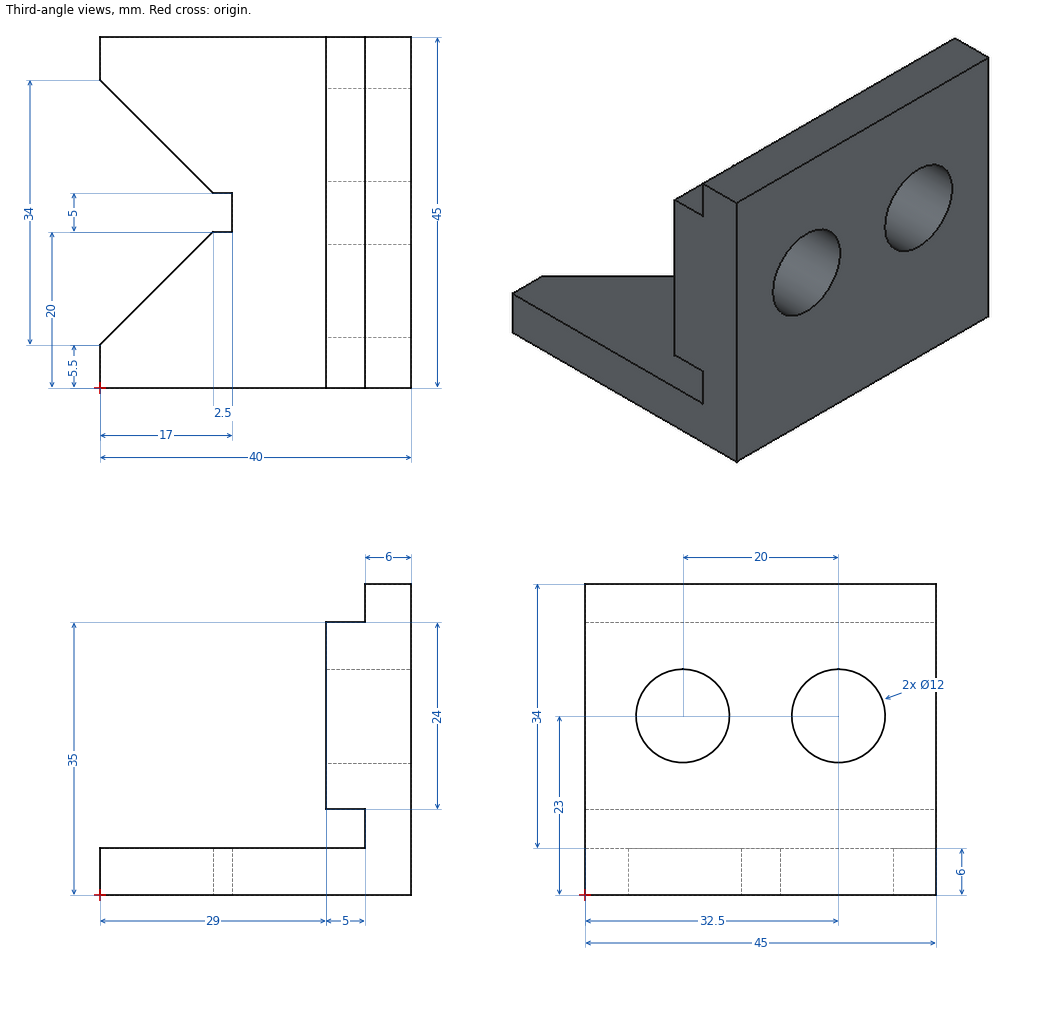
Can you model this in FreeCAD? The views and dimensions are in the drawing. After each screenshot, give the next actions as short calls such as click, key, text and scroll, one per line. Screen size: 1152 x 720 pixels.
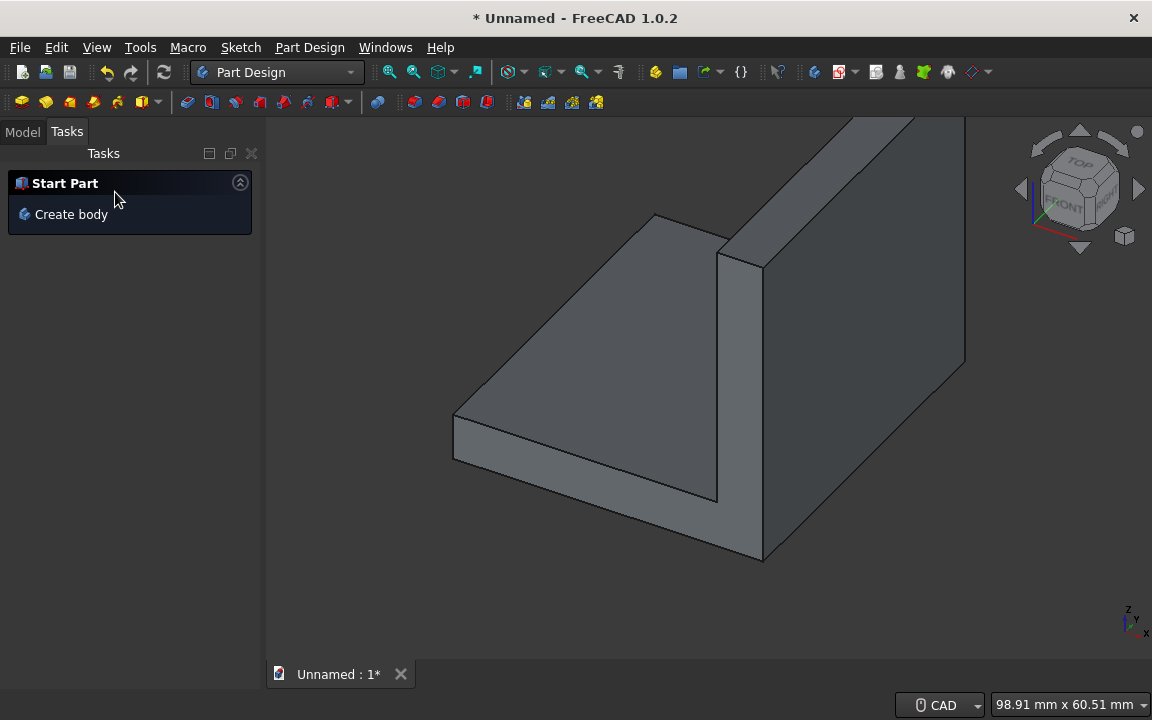
click(390, 72)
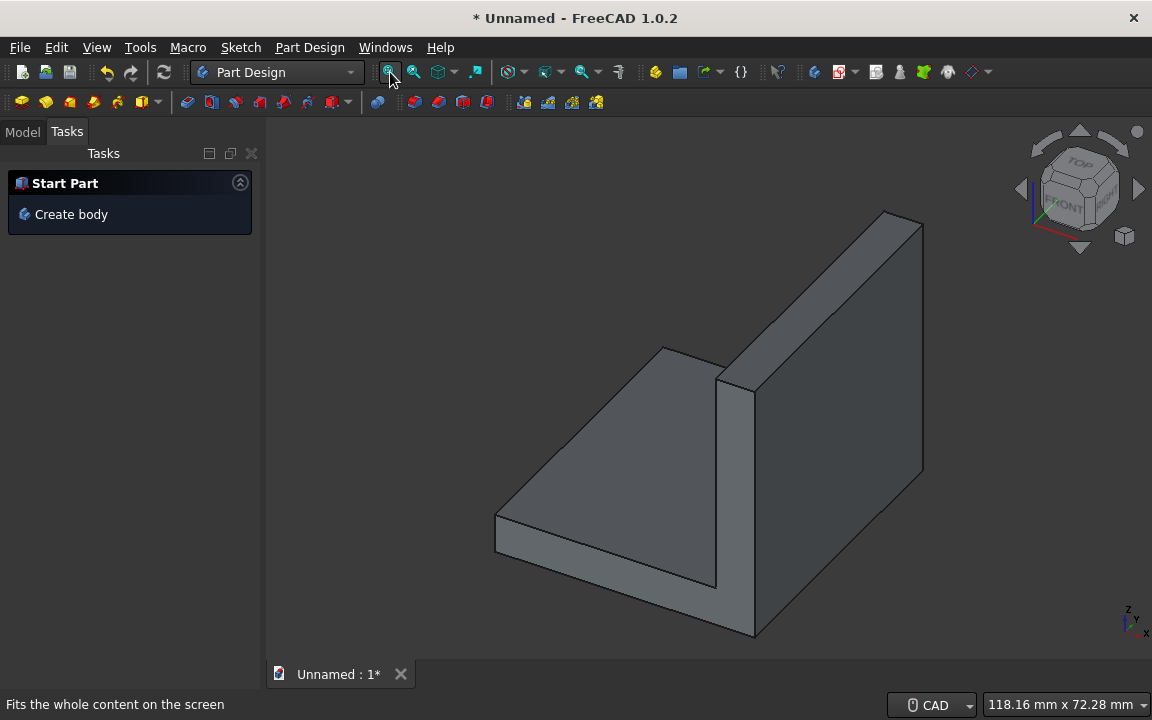
click(840, 72)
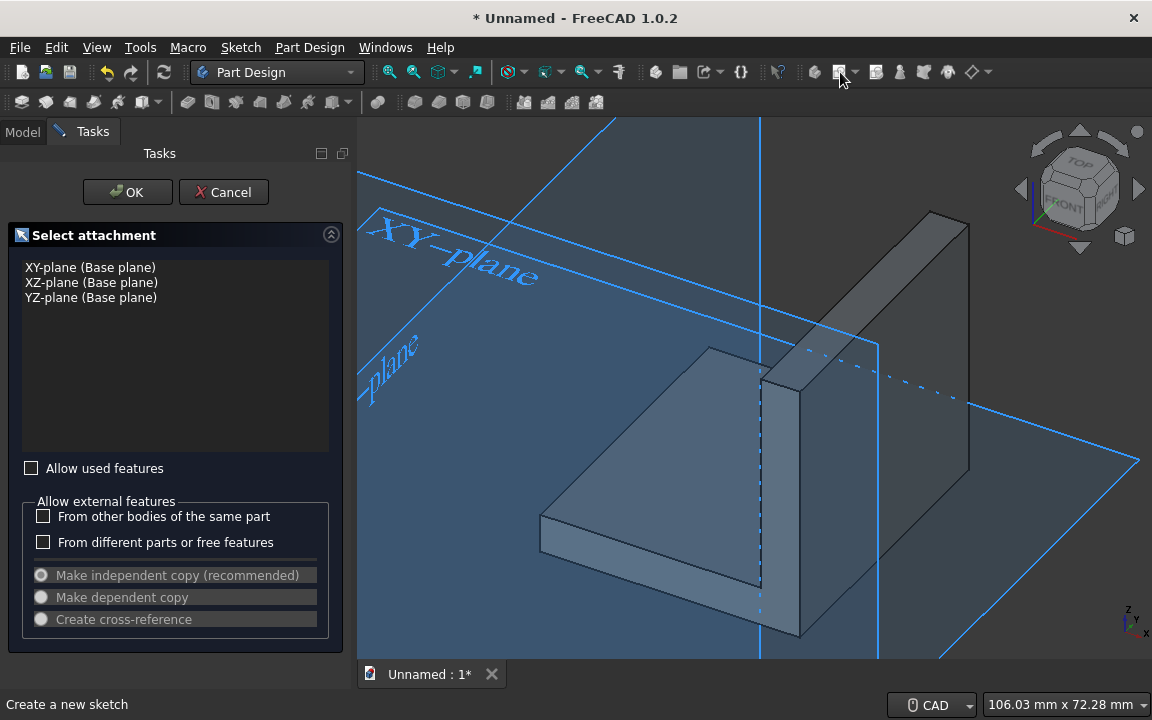
click(82, 282)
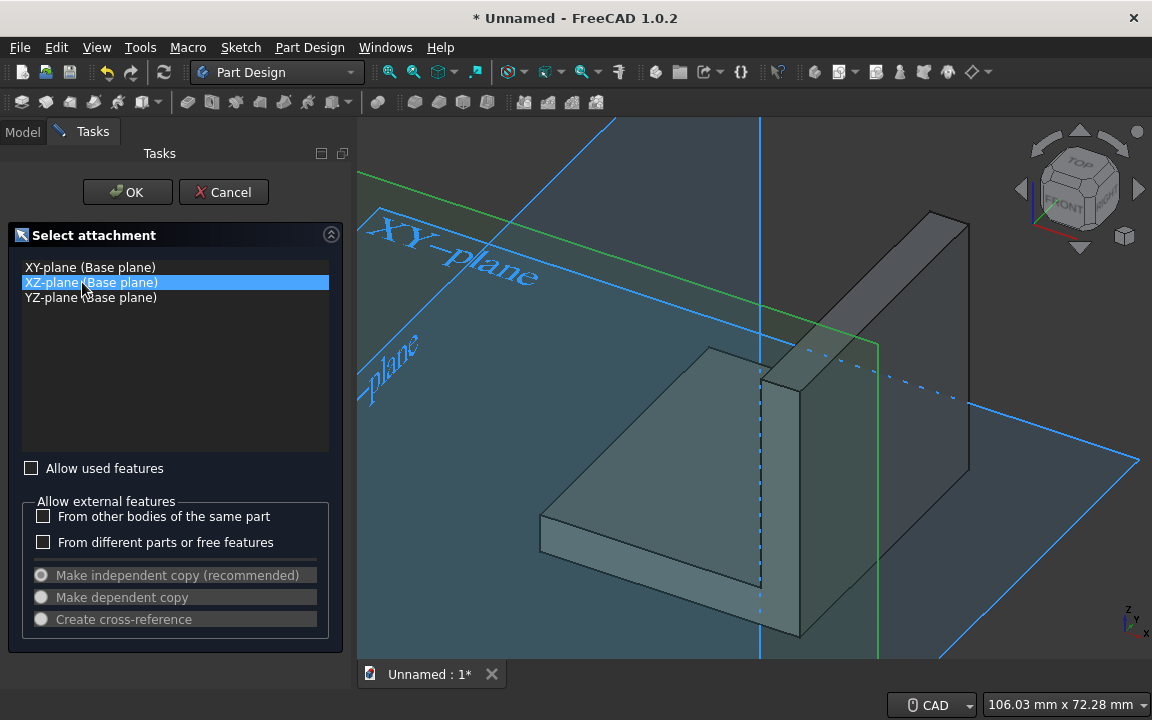
click(128, 192)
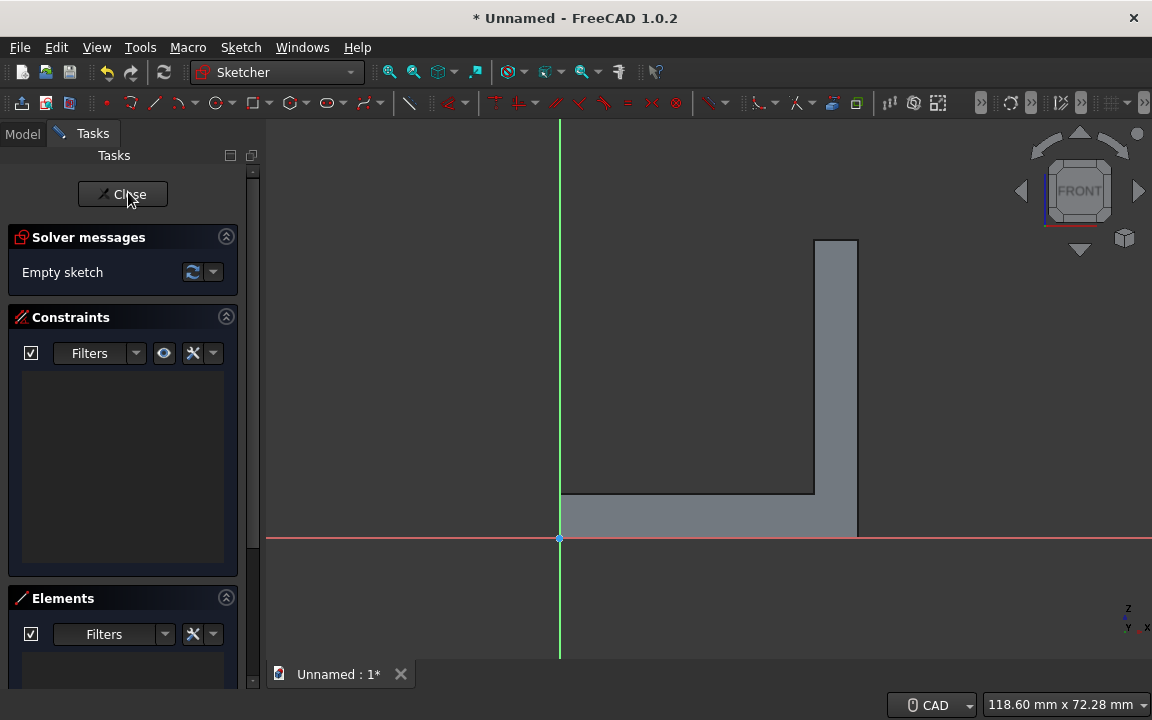
click(254, 104)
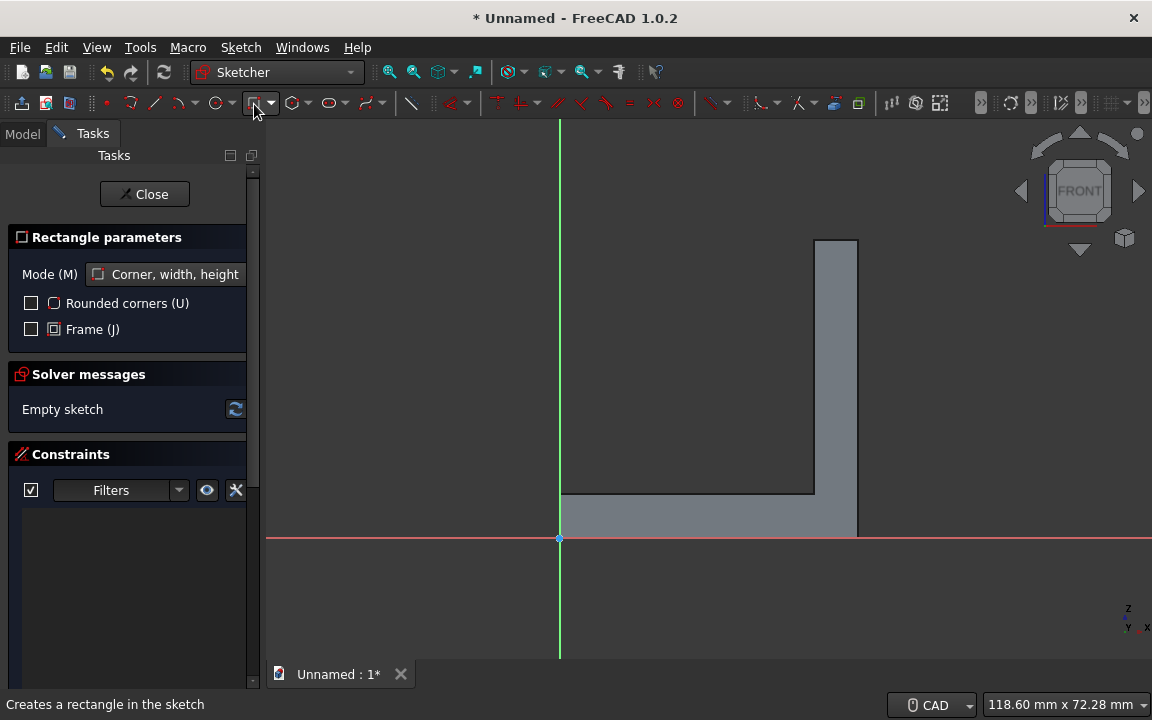
click(776, 277)
click(814, 456)
key(Escape)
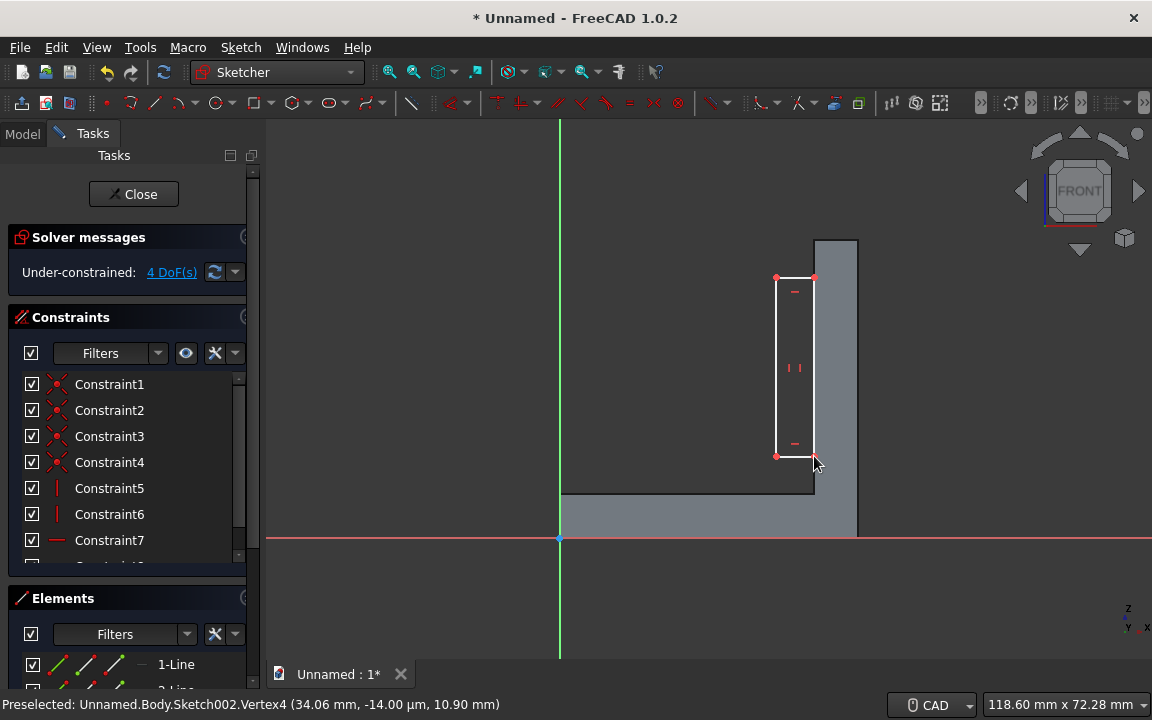
click(450, 104)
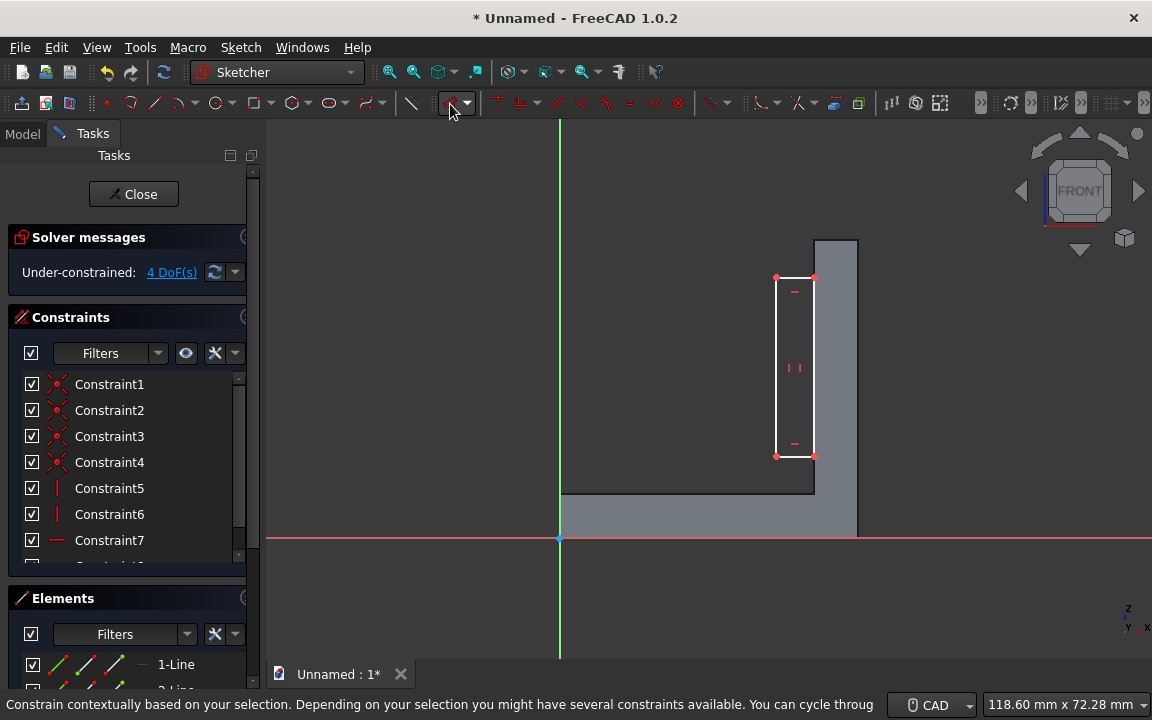
click(787, 457)
click(795, 491)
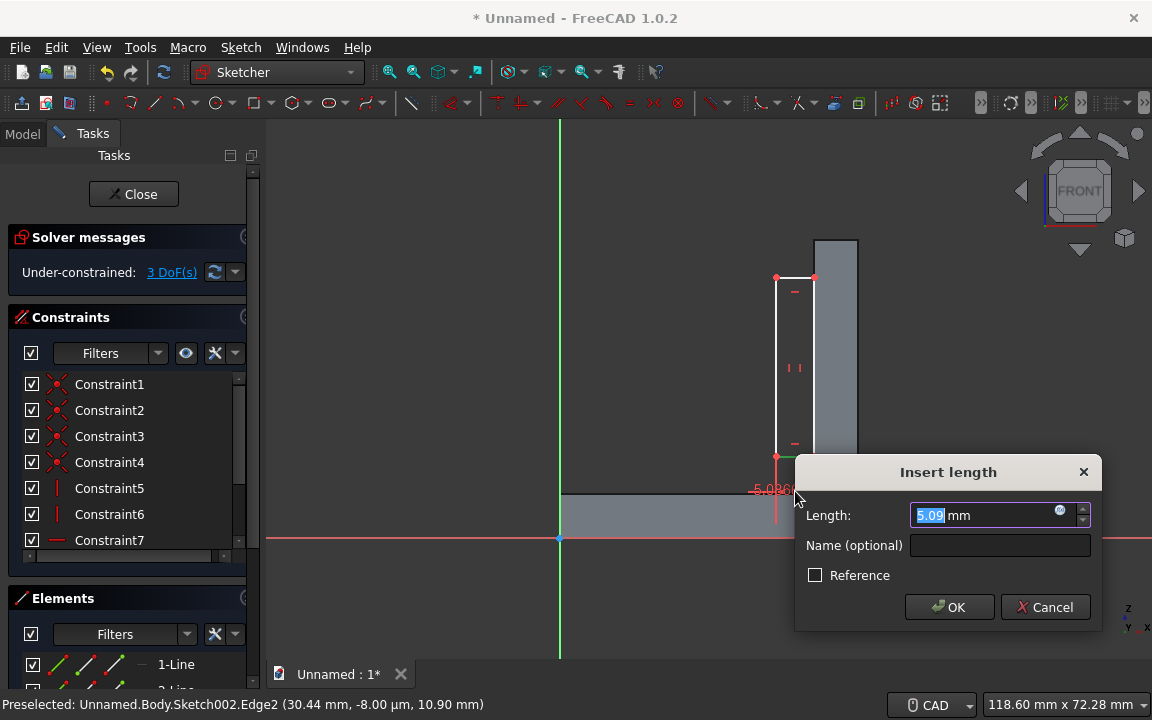
text(5)
key(Return)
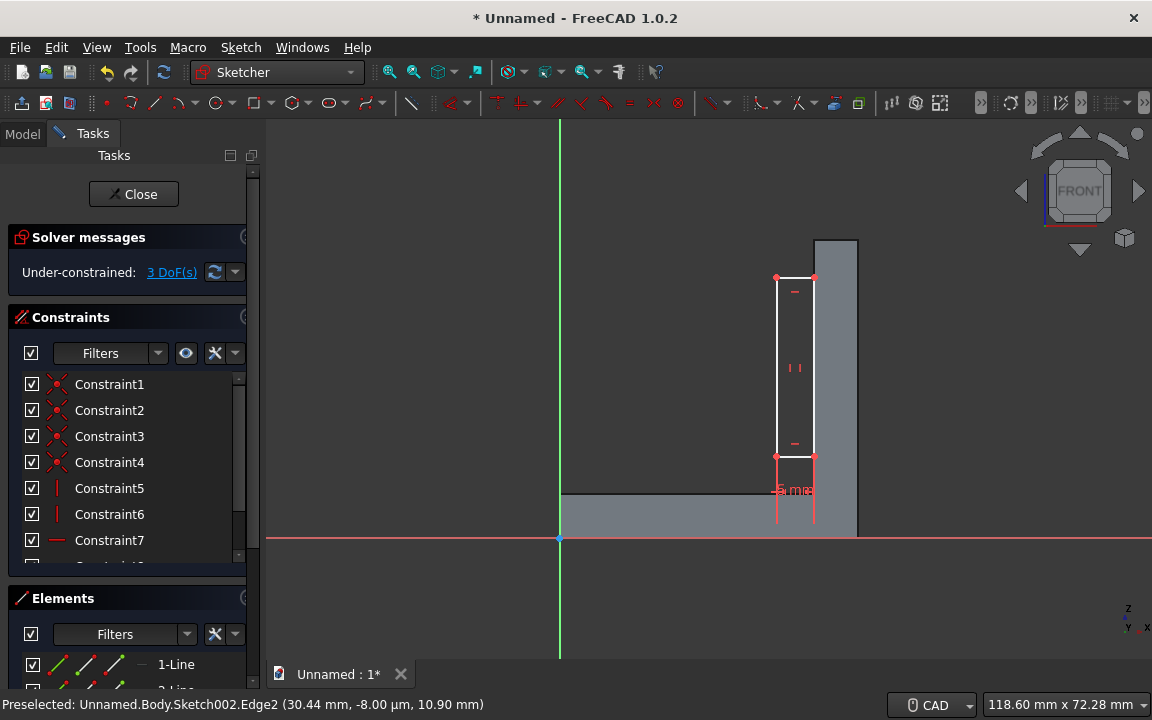
click(777, 332)
click(743, 368)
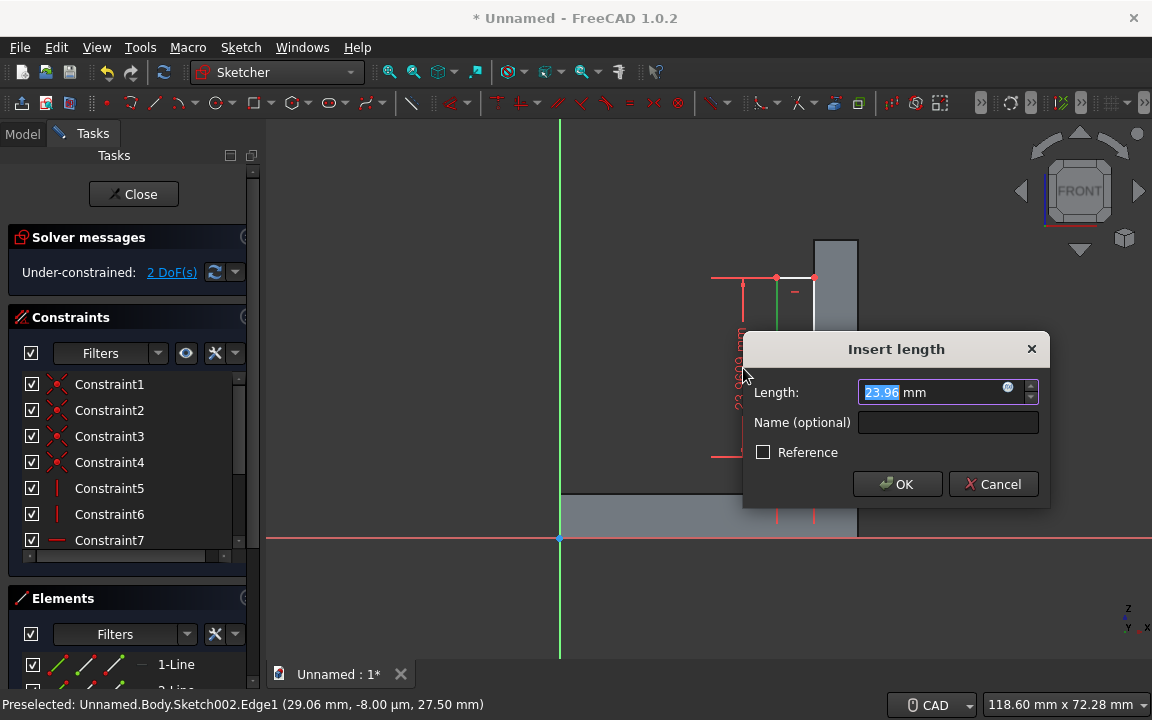
text(24)
key(Return)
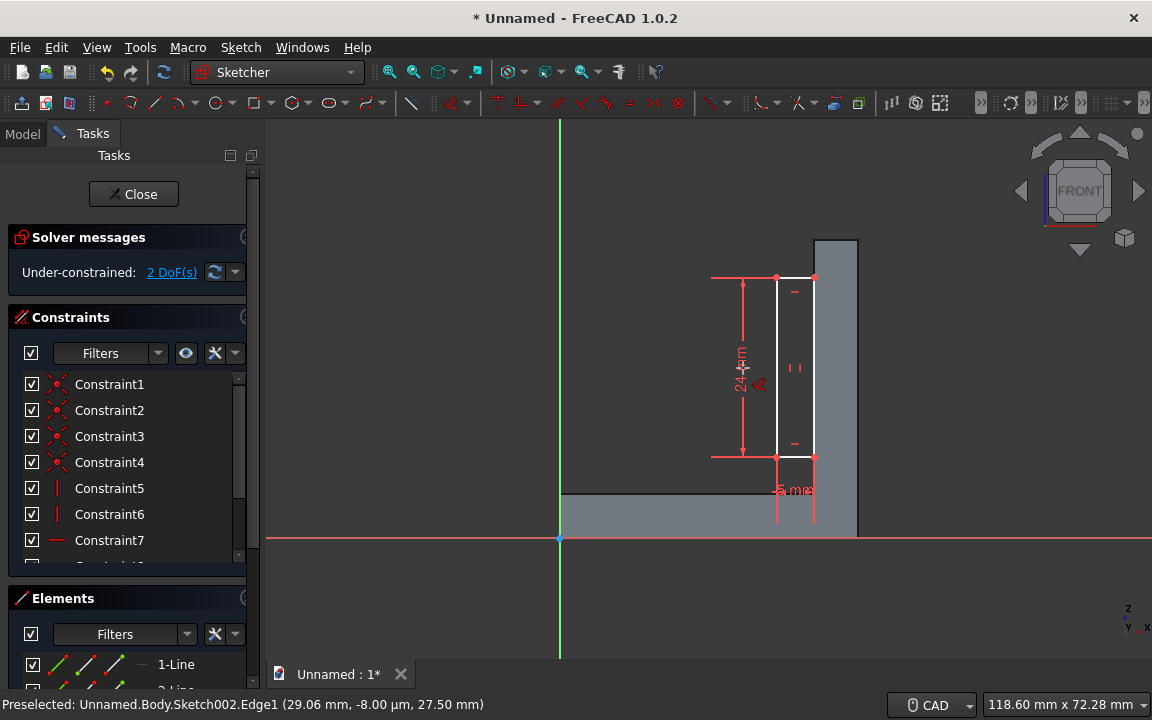
click(777, 278)
click(668, 572)